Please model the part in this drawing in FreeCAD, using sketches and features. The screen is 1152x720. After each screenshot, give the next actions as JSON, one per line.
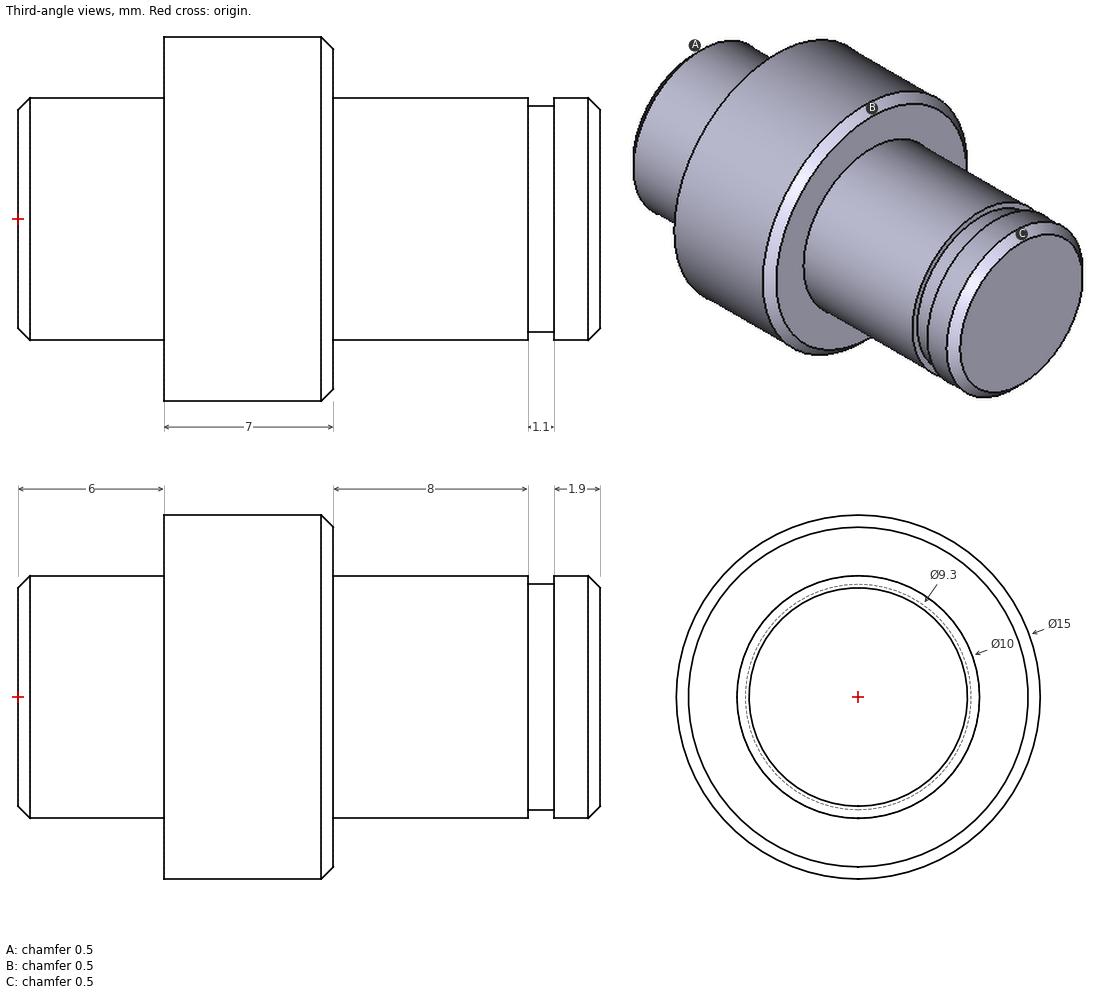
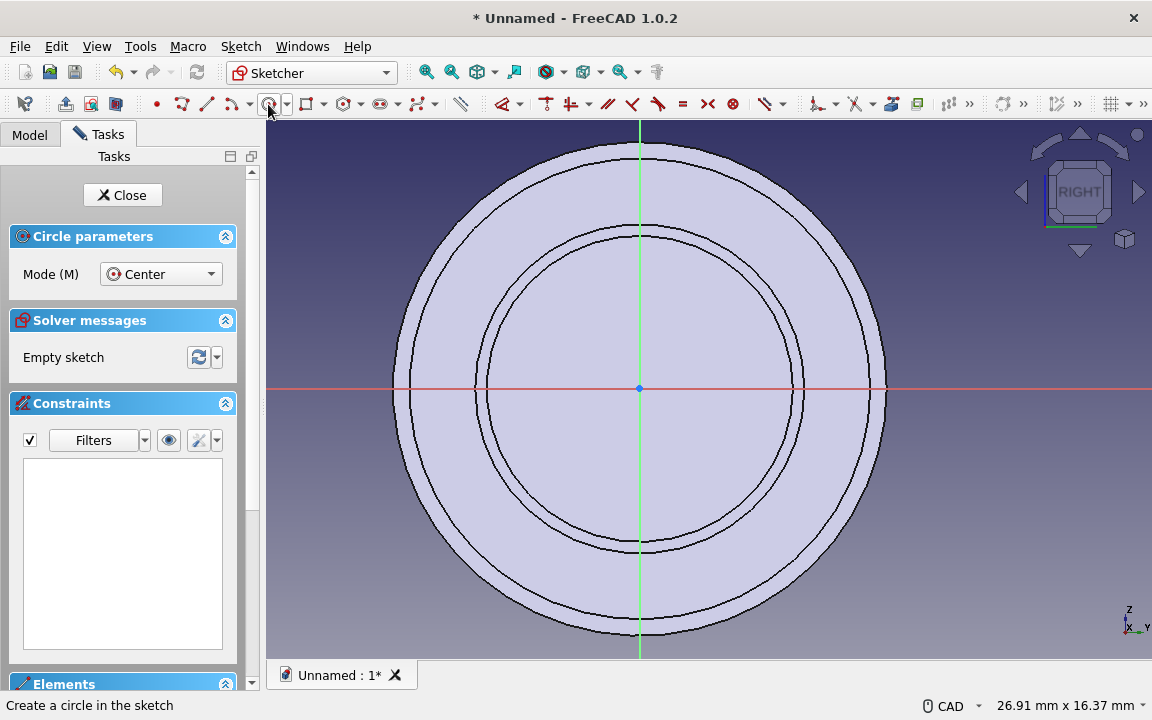
{"action": "left_click", "coordinate": [640, 389]}
{"action": "mouse_move", "coordinate": [756, 272]}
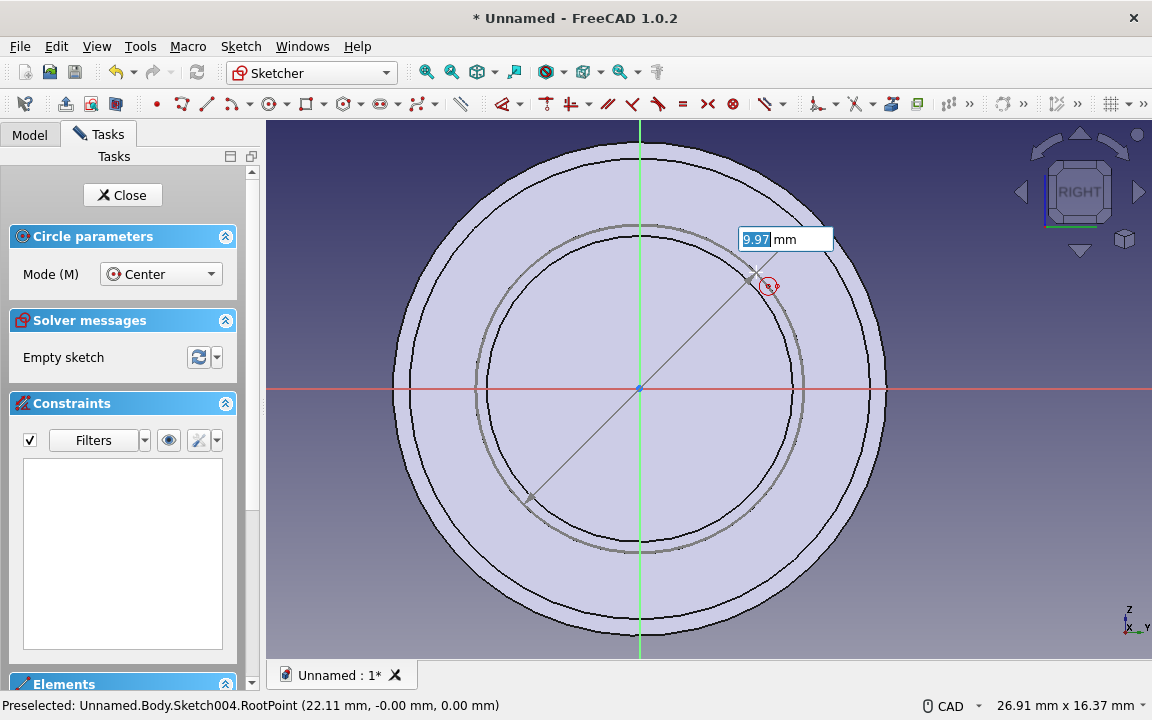
{"action": "type", "text": "10"}
{"action": "key", "text": "Return"}
{"action": "key", "text": "Escape"}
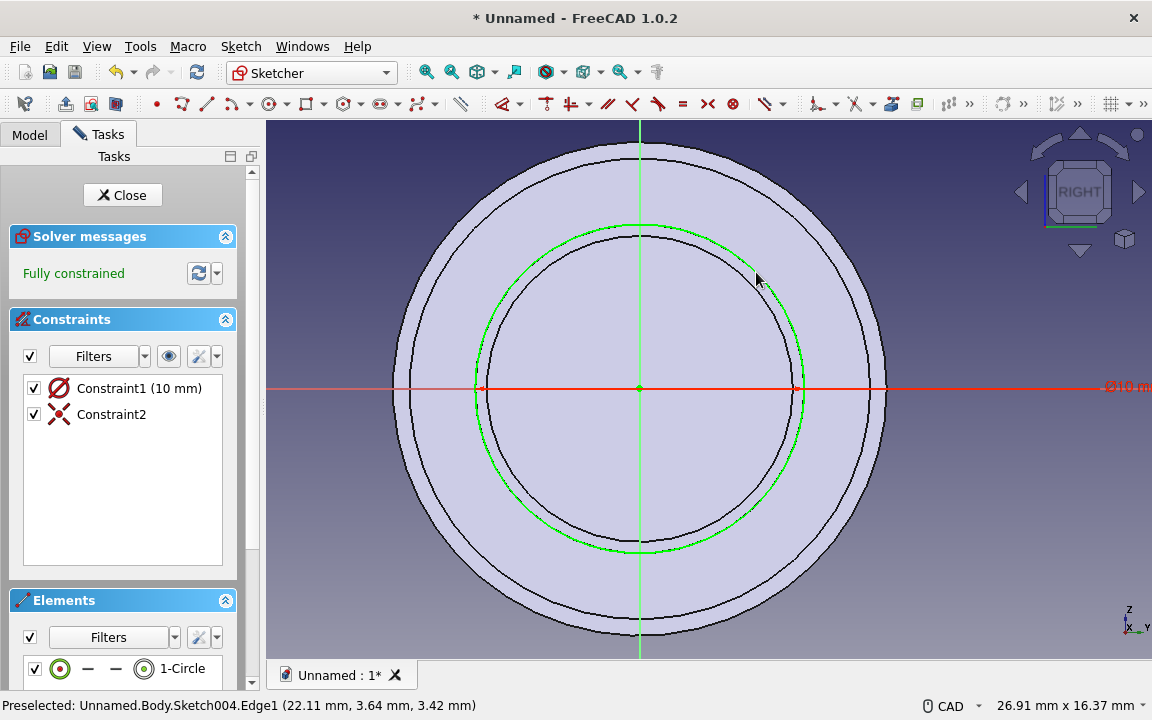
{"action": "left_click", "coordinate": [123, 195]}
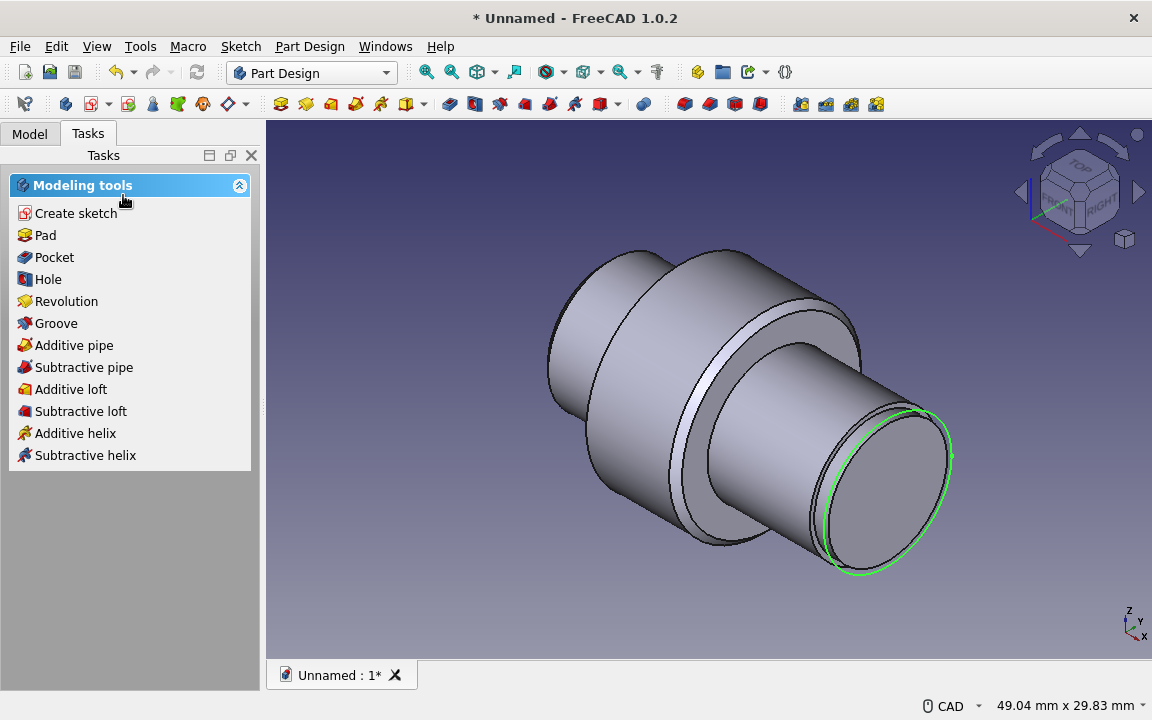
{"action": "left_click", "coordinate": [281, 104]}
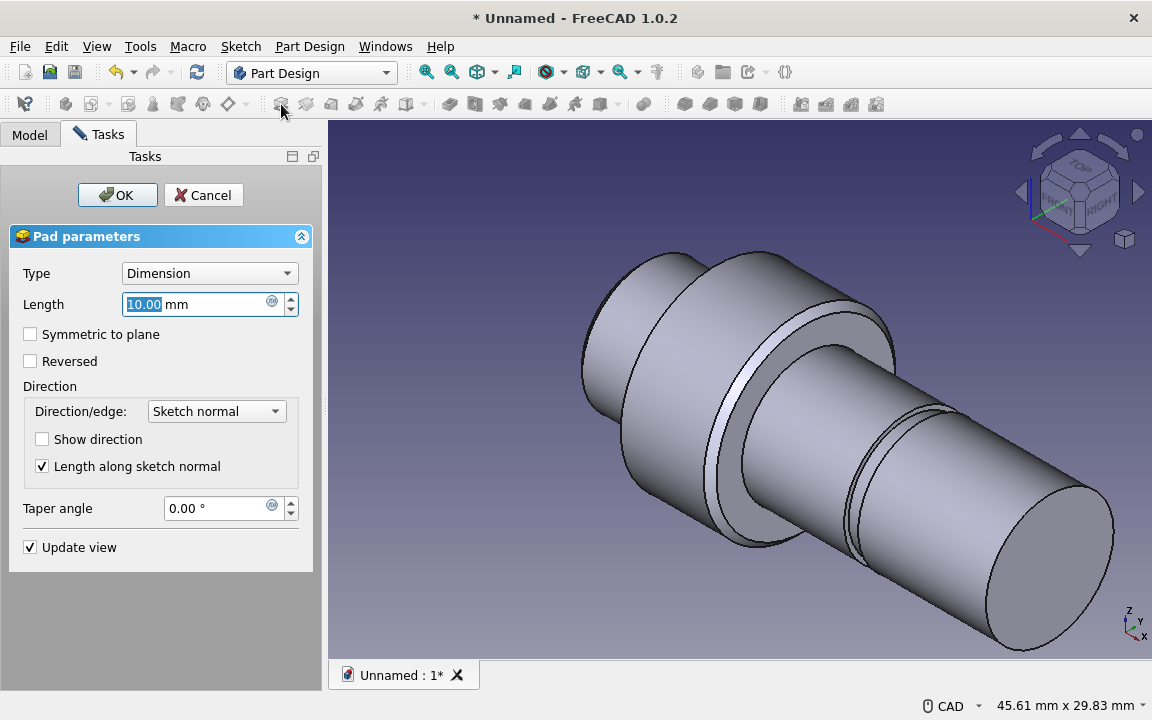
{"action": "type", "text": "1.9"}
{"action": "key", "text": "Tab"}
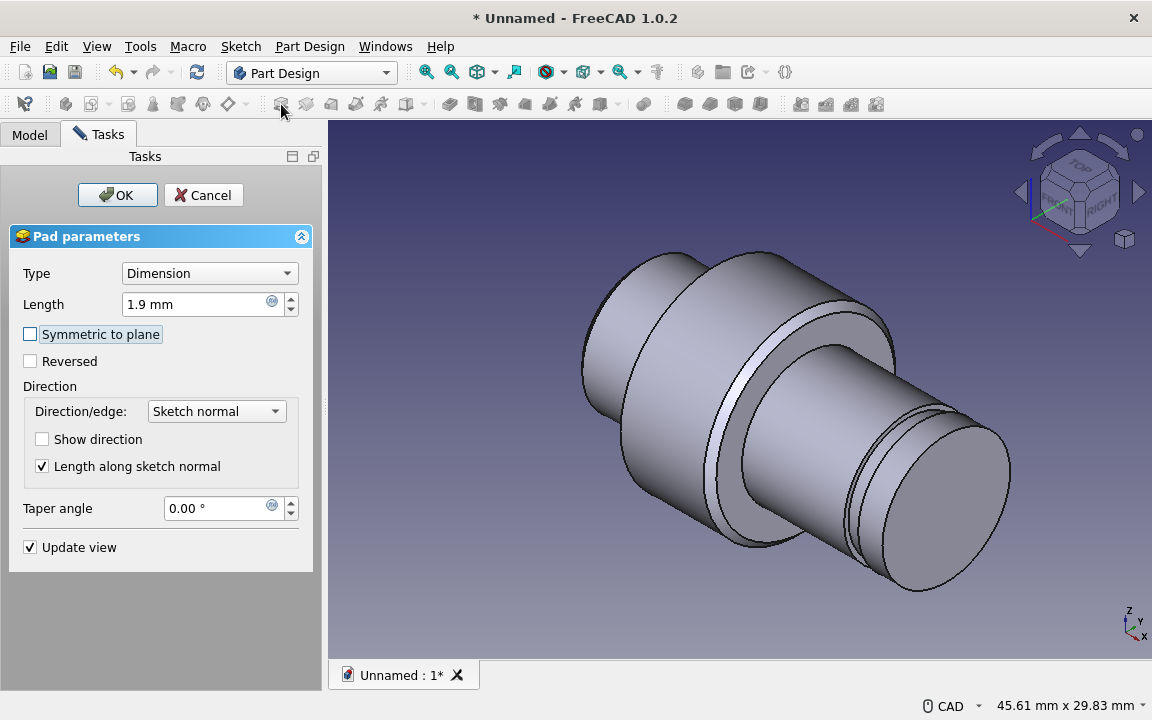
{"action": "left_click", "coordinate": [118, 195]}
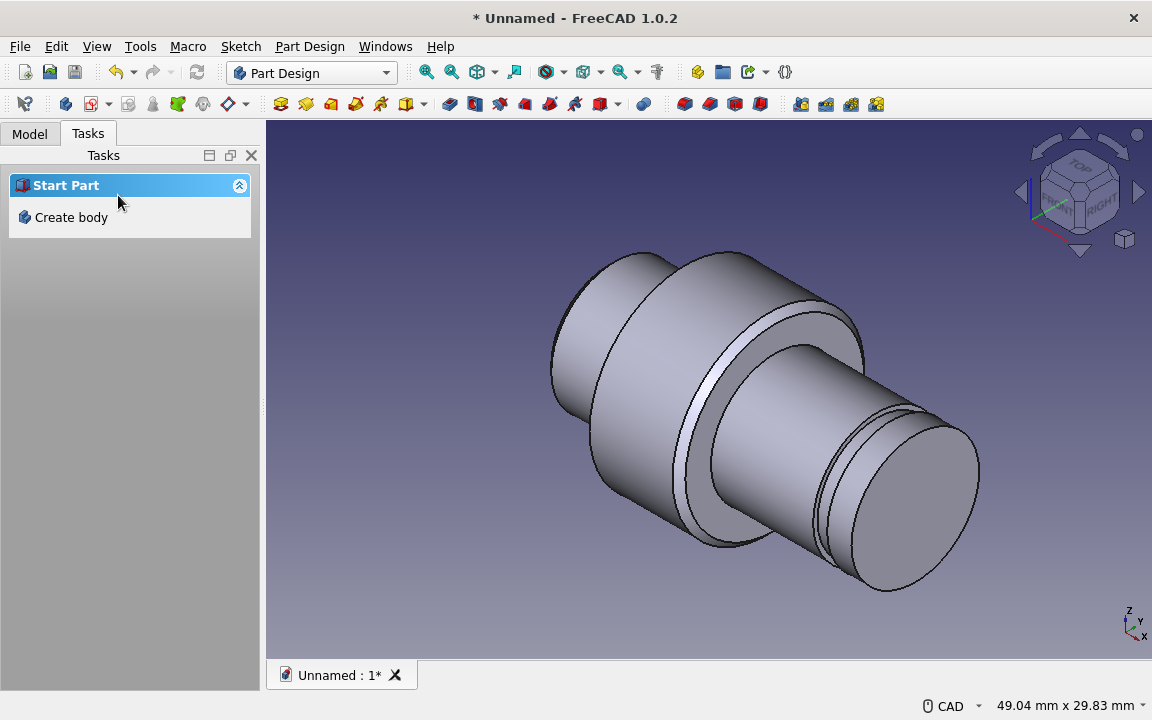
{"action": "key", "text": "v f"}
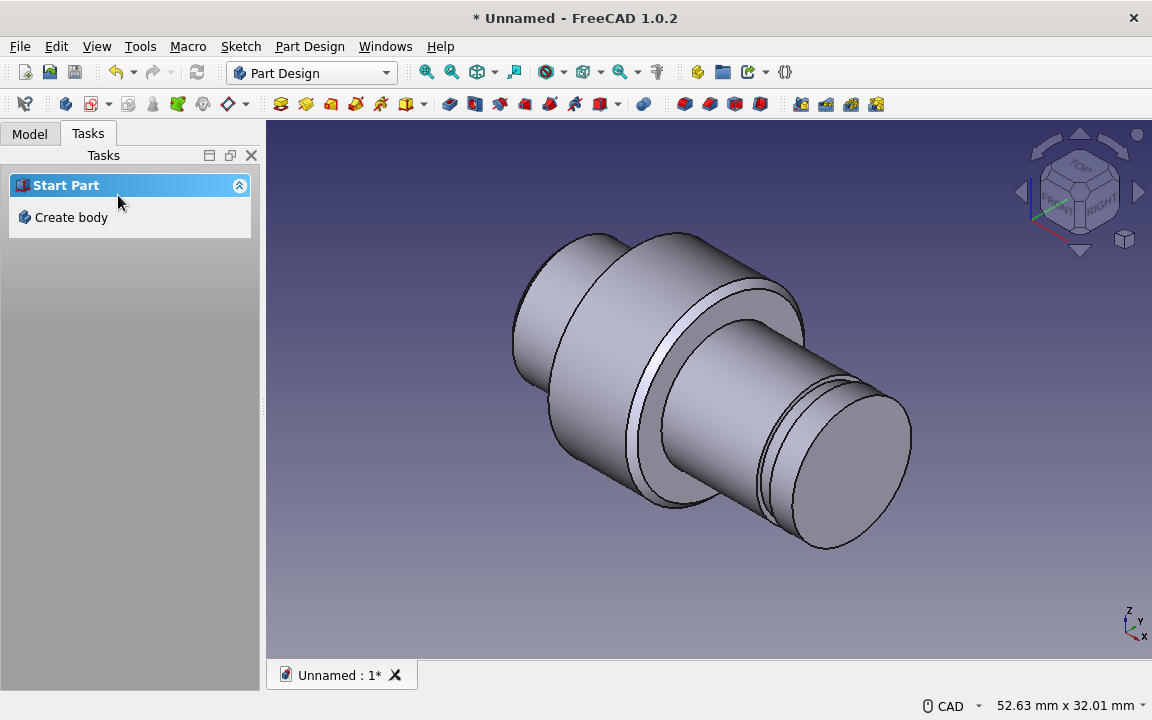
{"action": "left_click", "coordinate": [792, 505]}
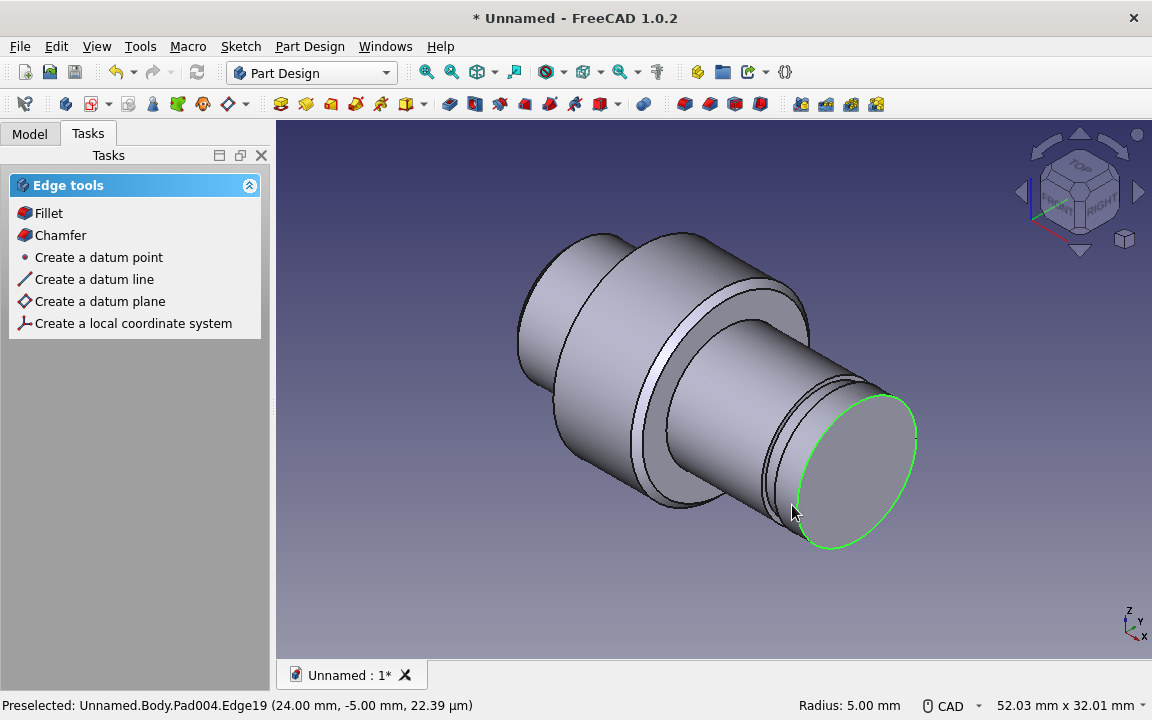
{"action": "left_click", "coordinate": [710, 104]}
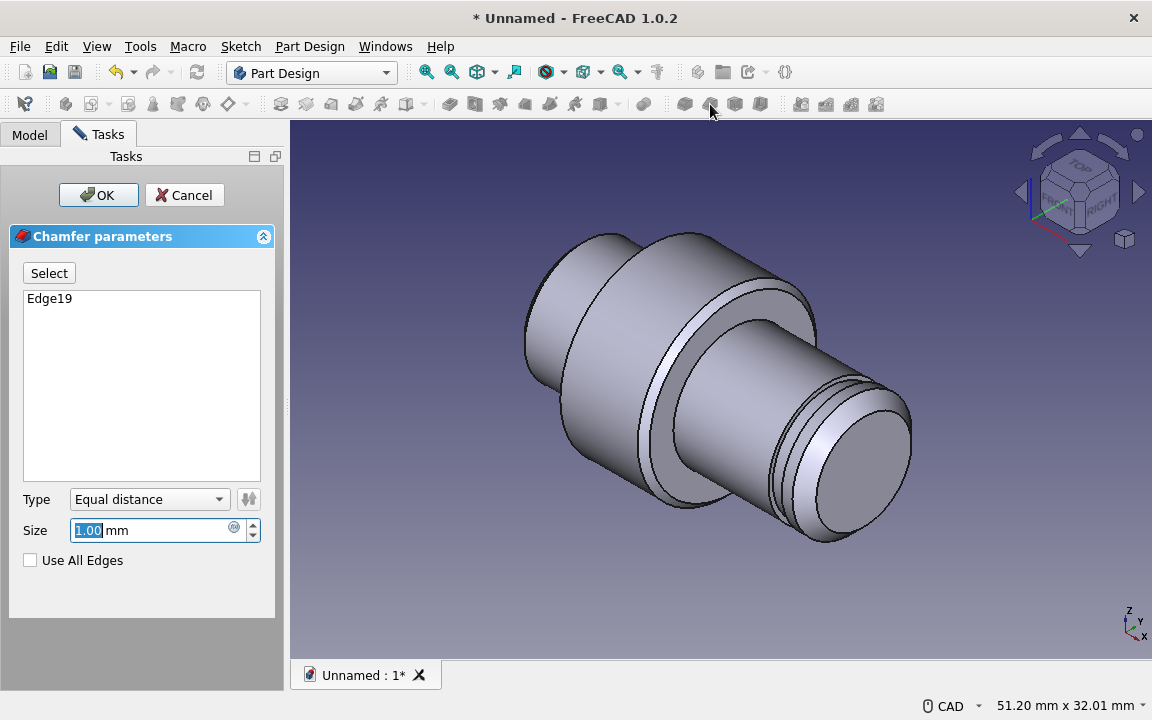
{"action": "type", "text": "0.5"}
{"action": "key", "text": "Tab"}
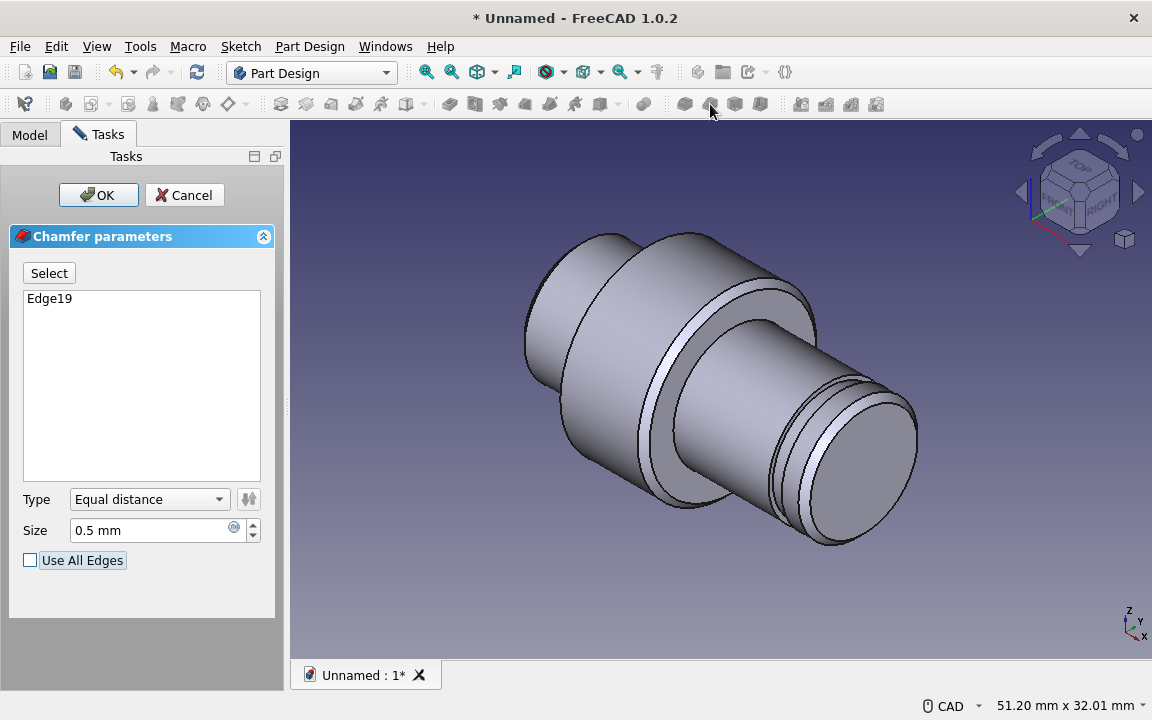
{"action": "left_click", "coordinate": [99, 195]}